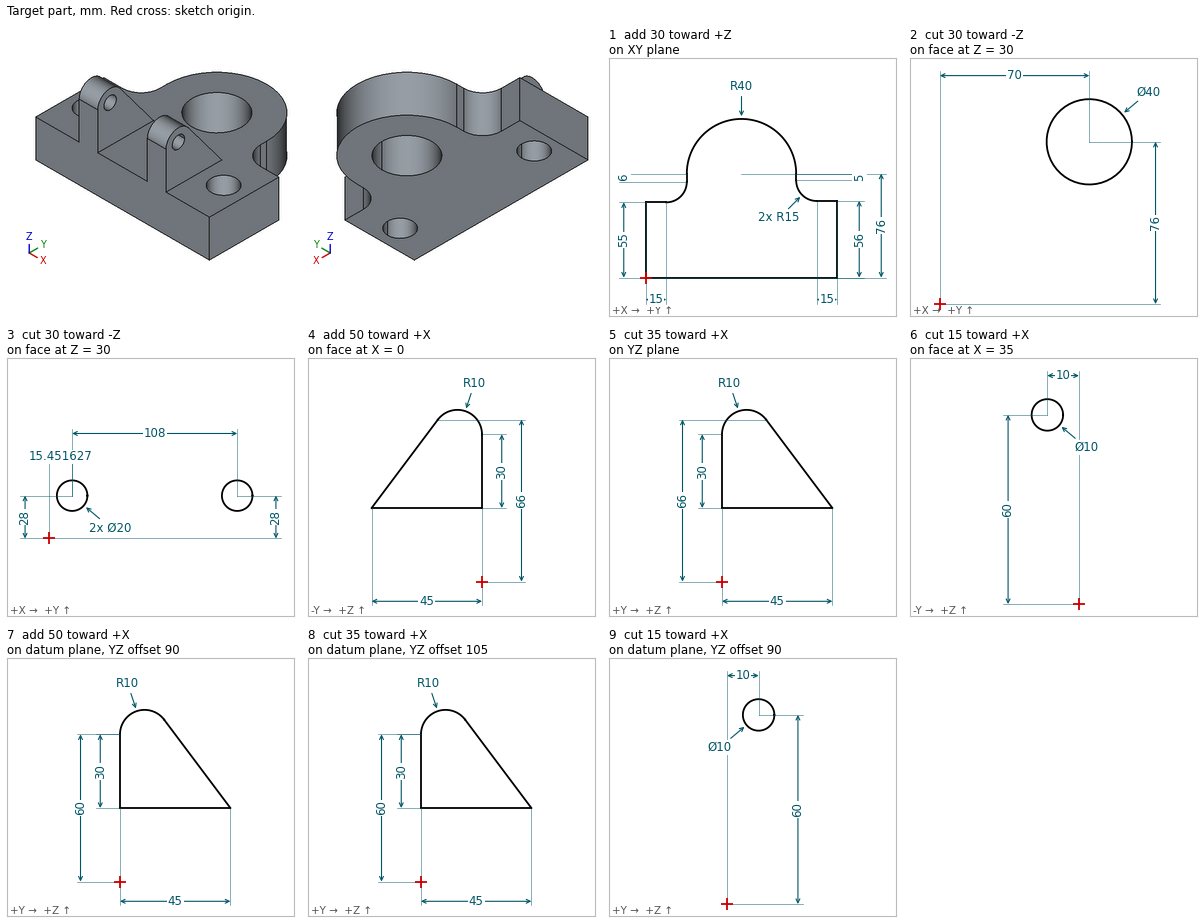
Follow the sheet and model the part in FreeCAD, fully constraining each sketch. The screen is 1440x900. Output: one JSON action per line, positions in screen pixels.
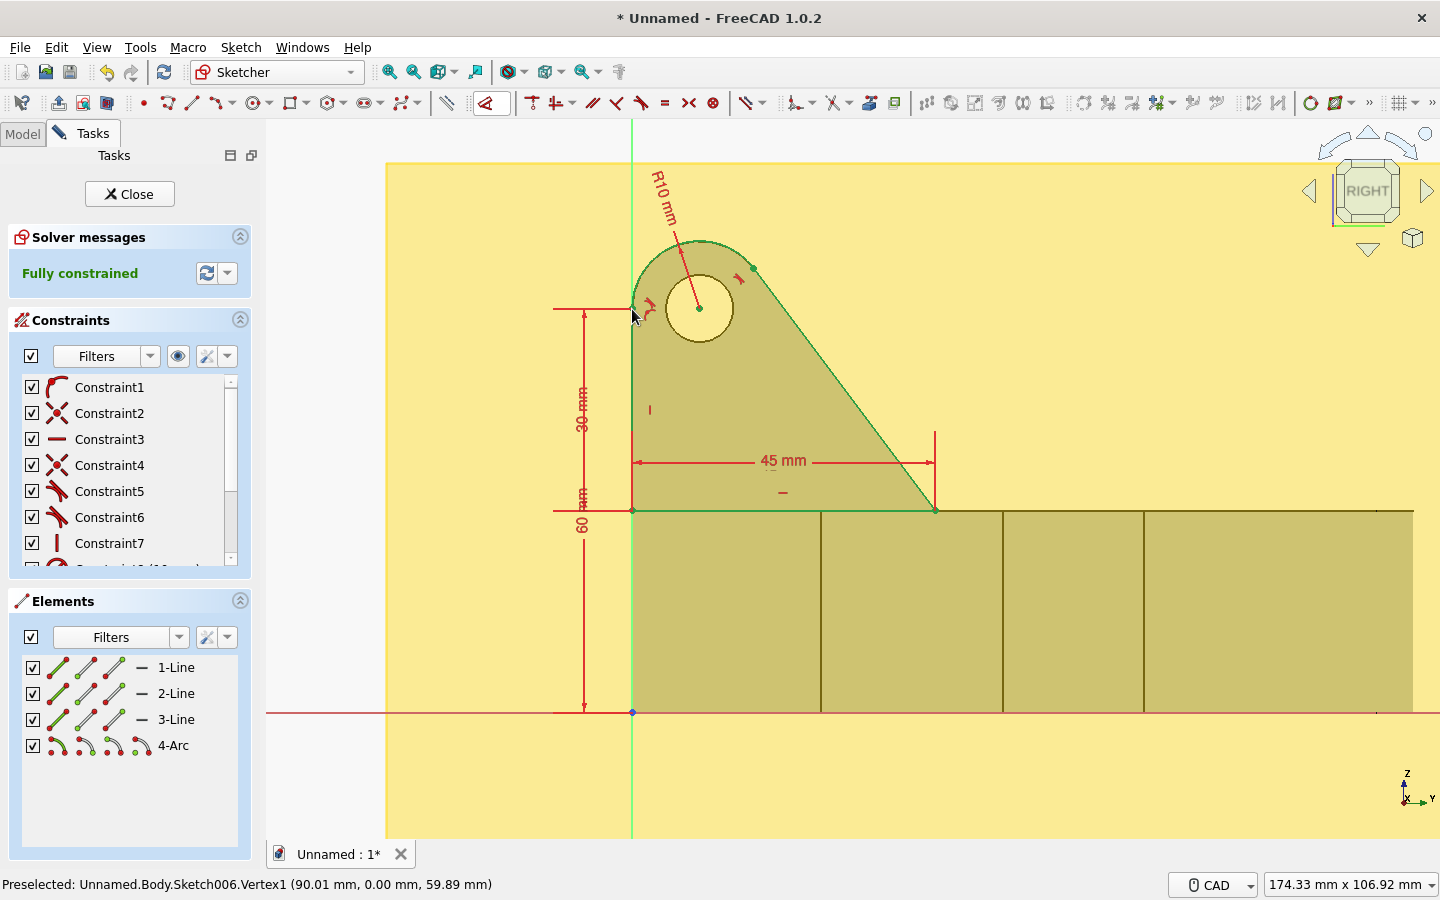
{"action": "left_click", "coordinate": [130, 194]}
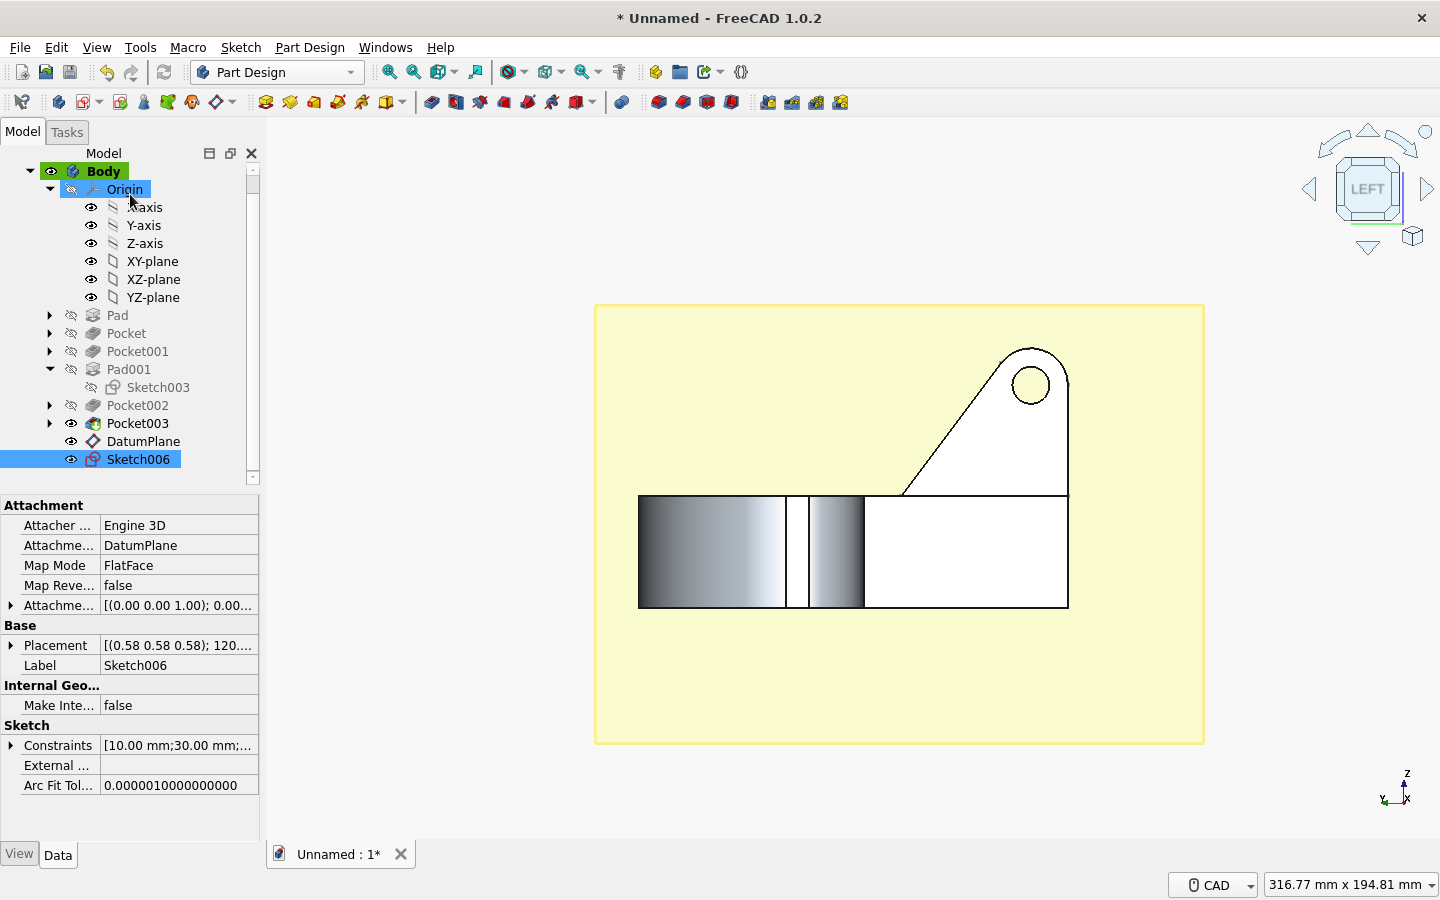
{"action": "left_click", "coordinate": [266, 102]}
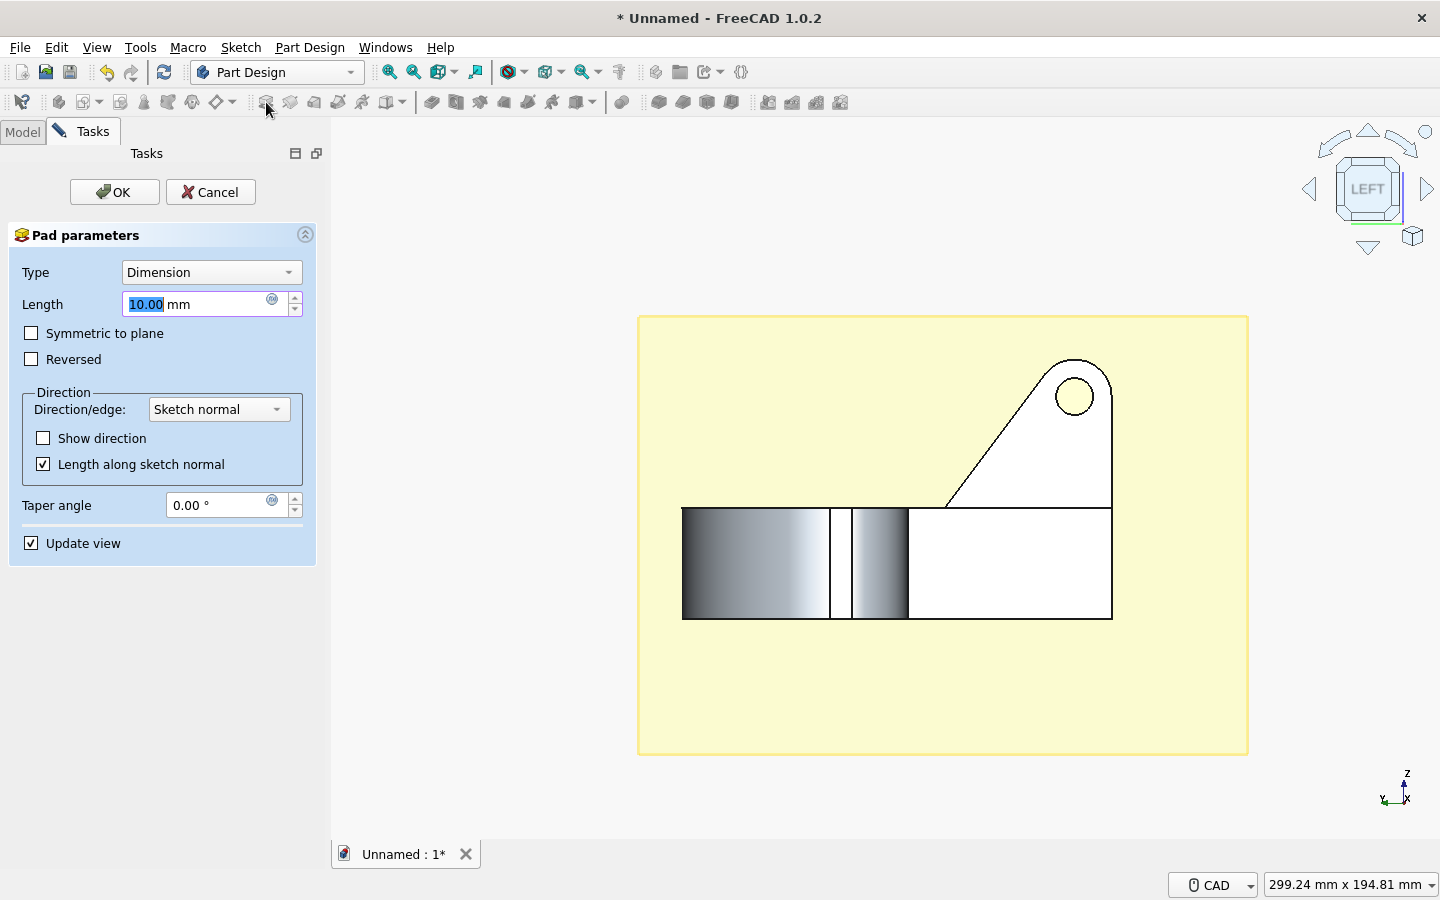
{"action": "type", "text": "50"}
{"action": "key", "text": "Tab"}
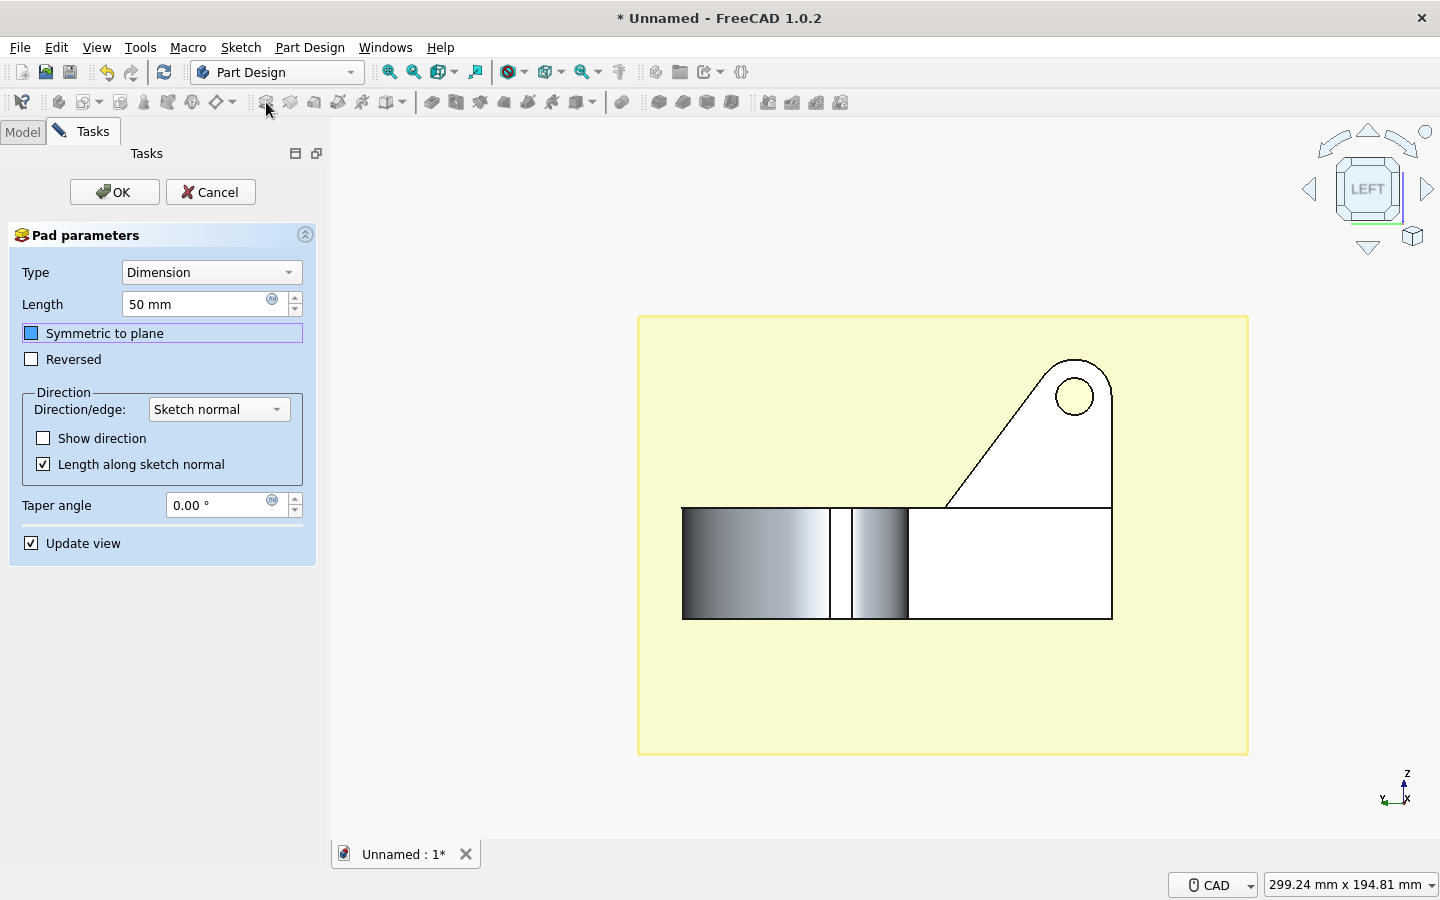
{"action": "left_click", "coordinate": [115, 192]}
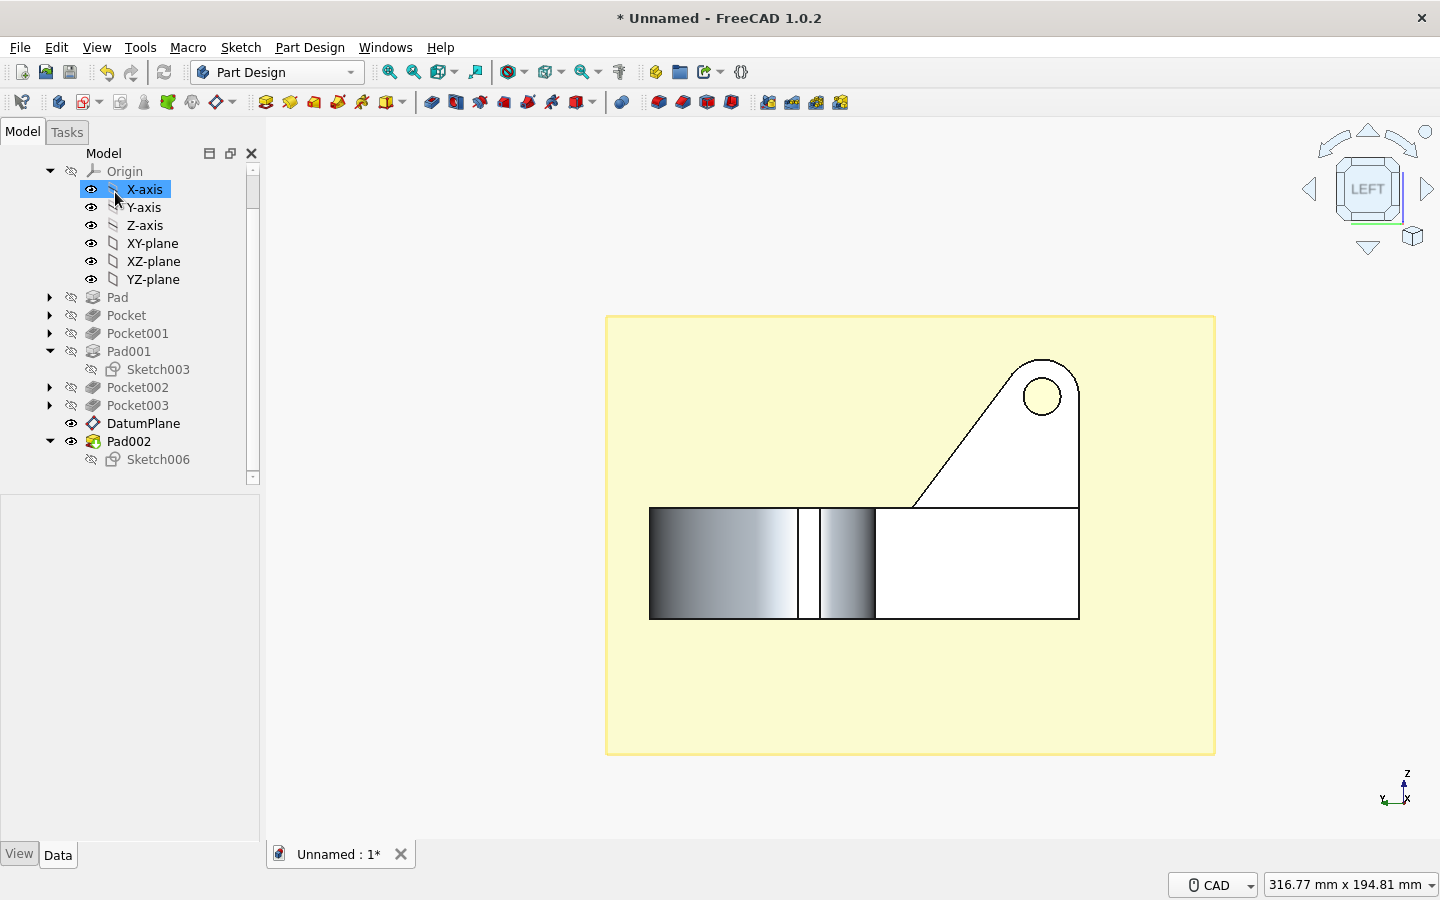
{"action": "left_click", "coordinate": [116, 423]}
{"action": "key", "text": "space"}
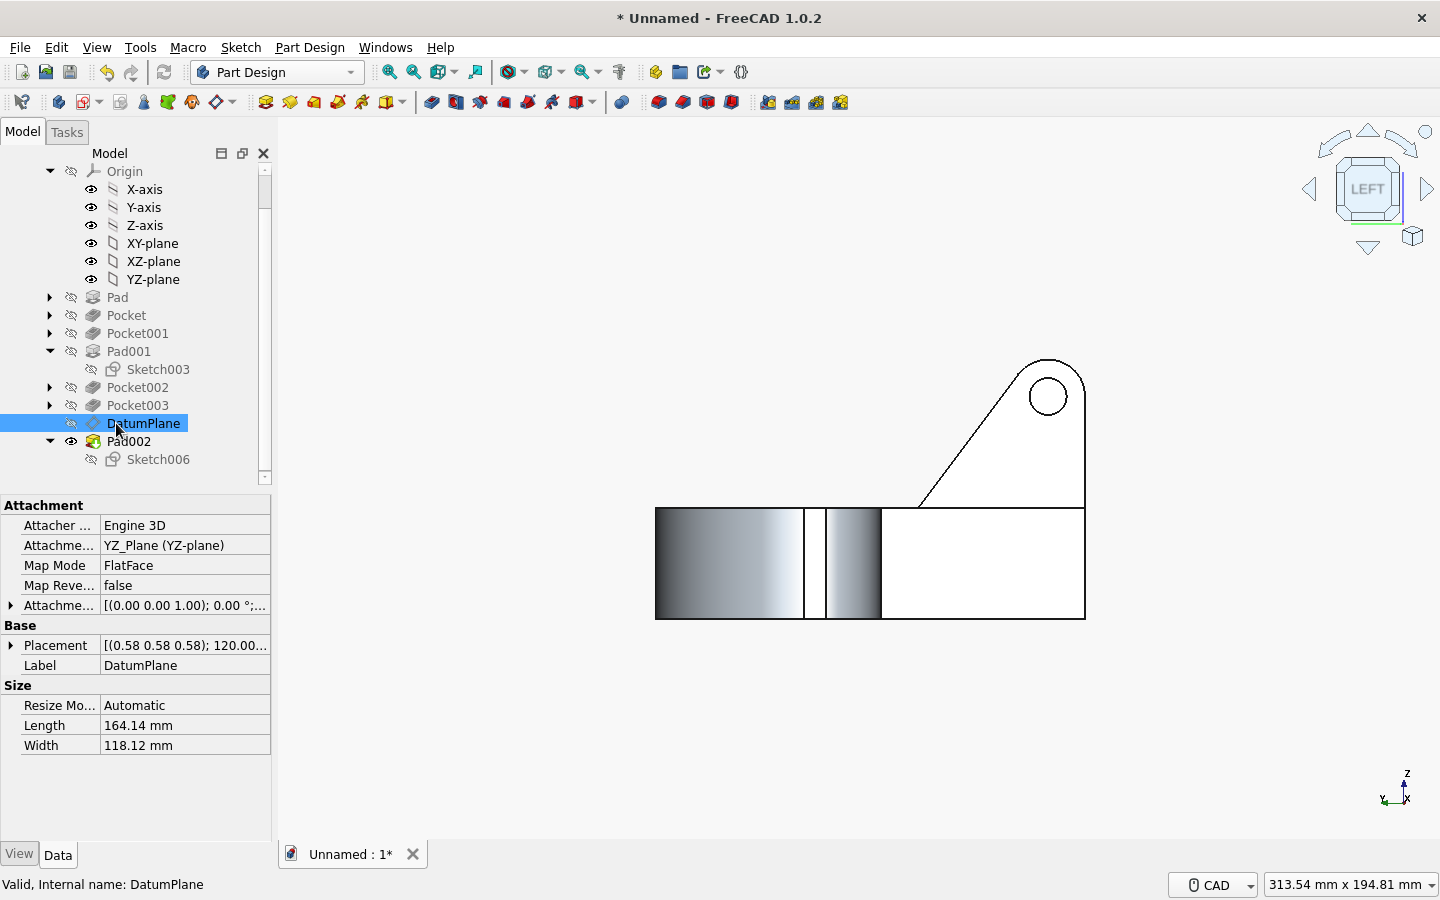
{"action": "key", "text": "v f"}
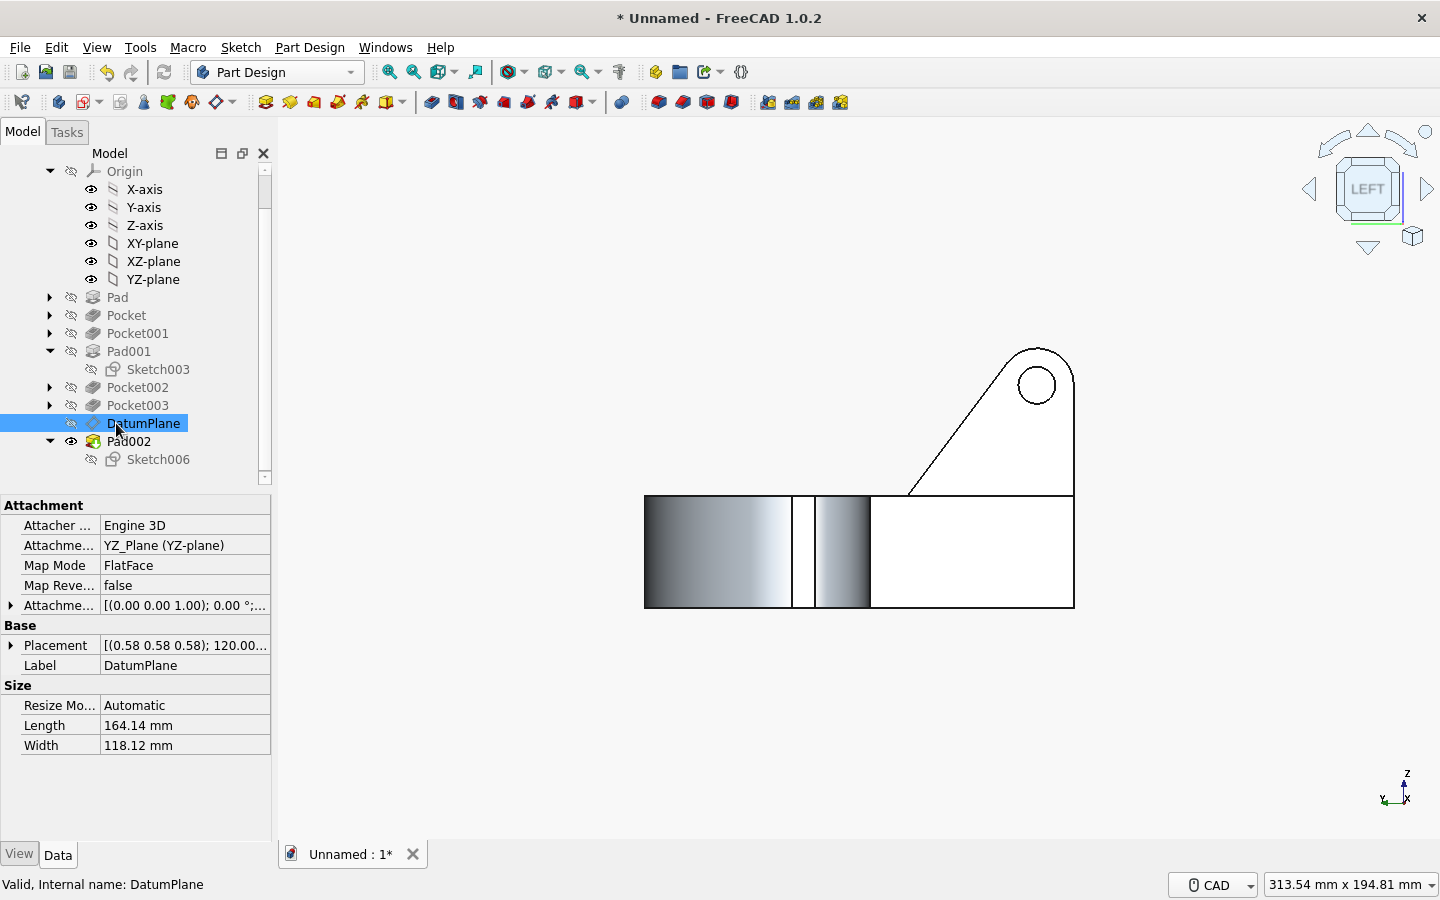
{"action": "left_click", "coordinate": [136, 279]}